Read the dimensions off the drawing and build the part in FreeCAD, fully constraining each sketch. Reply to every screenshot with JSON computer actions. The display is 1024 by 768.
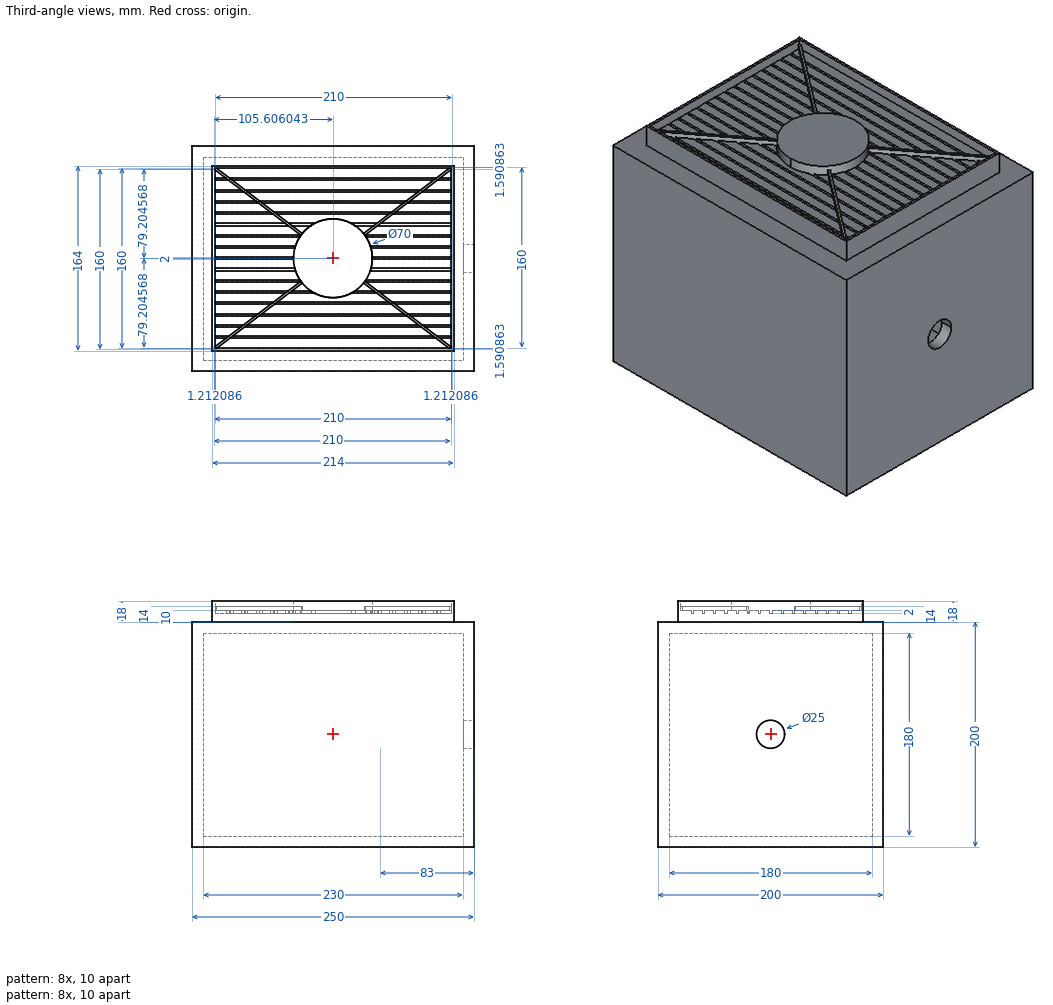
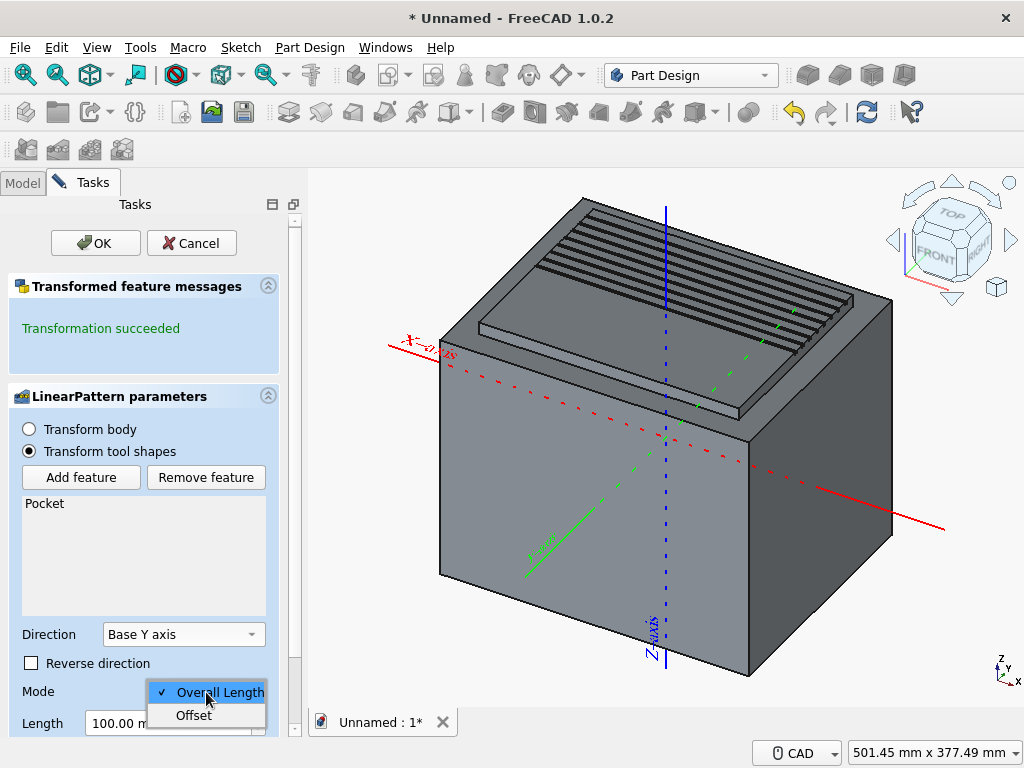
{"action": "left_click", "coordinate": [206, 716]}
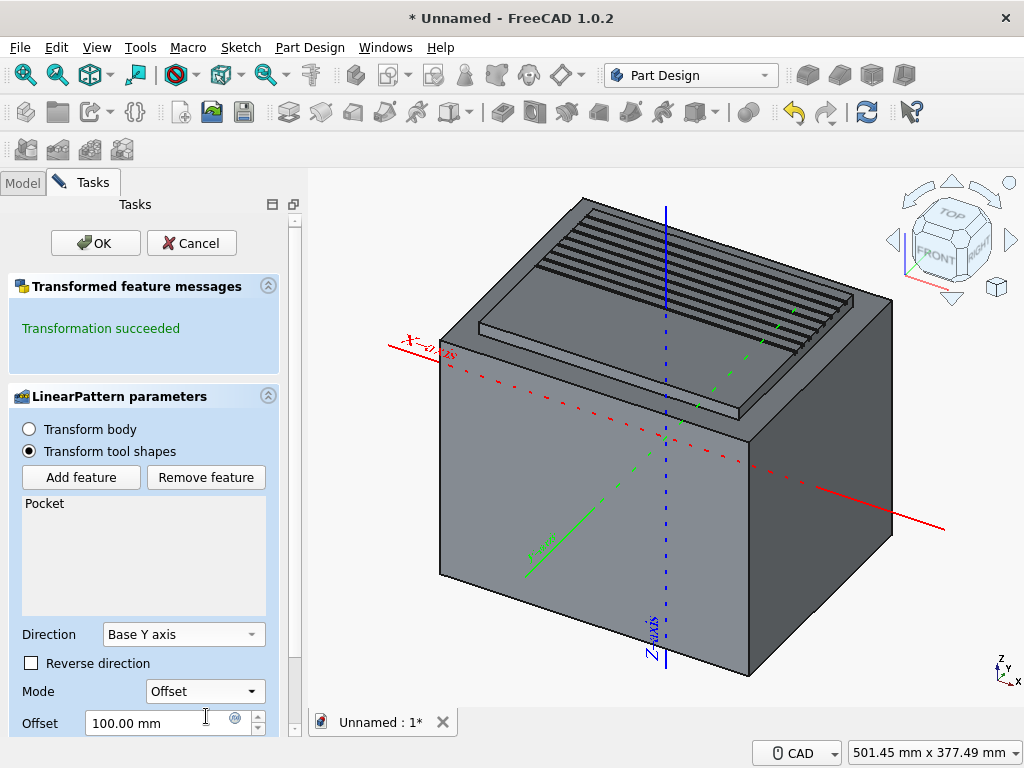
{"action": "triple_click", "coordinate": [168, 723]}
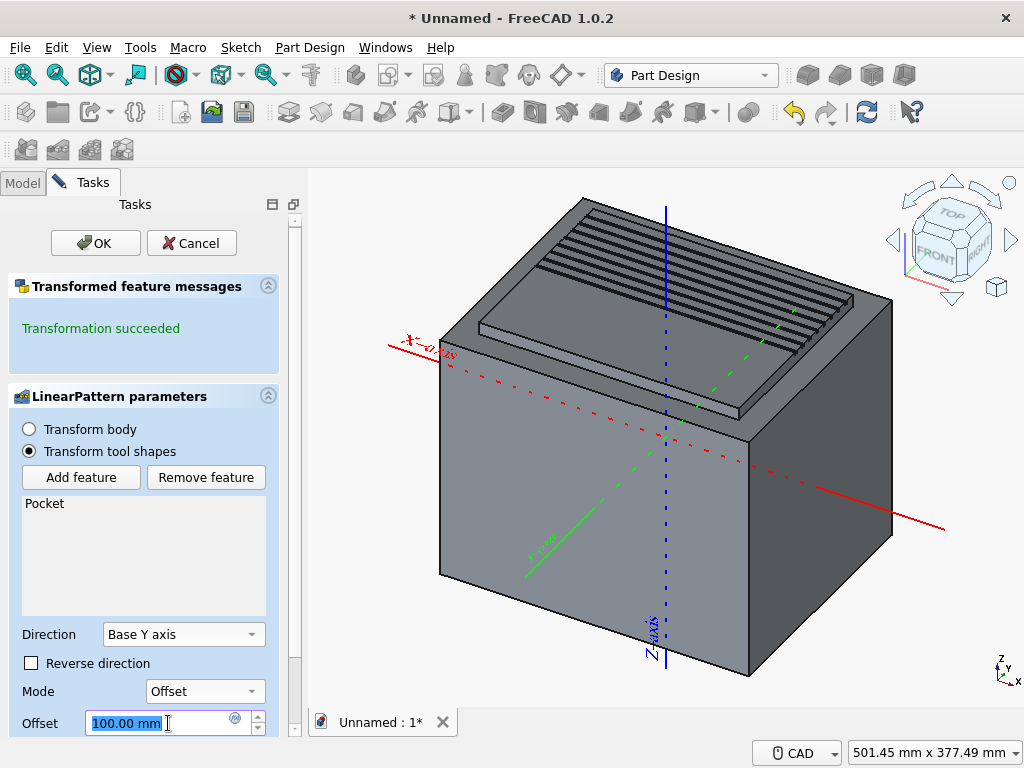
{"action": "type", "text": "10"}
{"action": "key", "text": "Tab"}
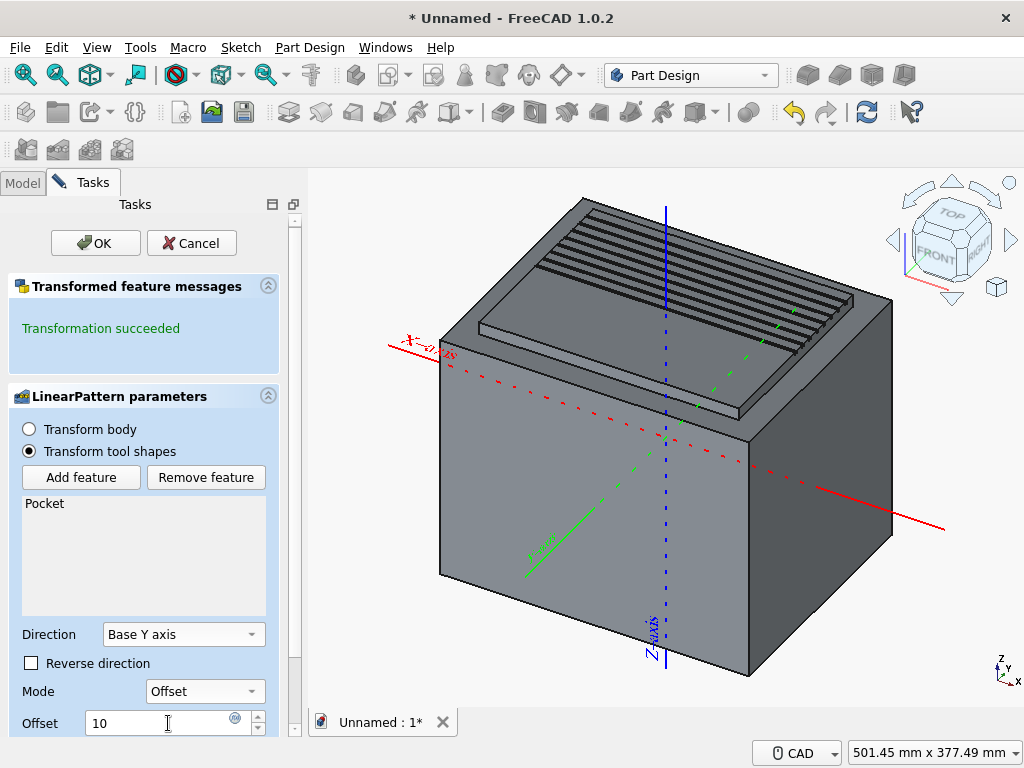
{"action": "scroll", "coordinate": [295, 475], "scroll_direction": "down", "scroll_amount": 2}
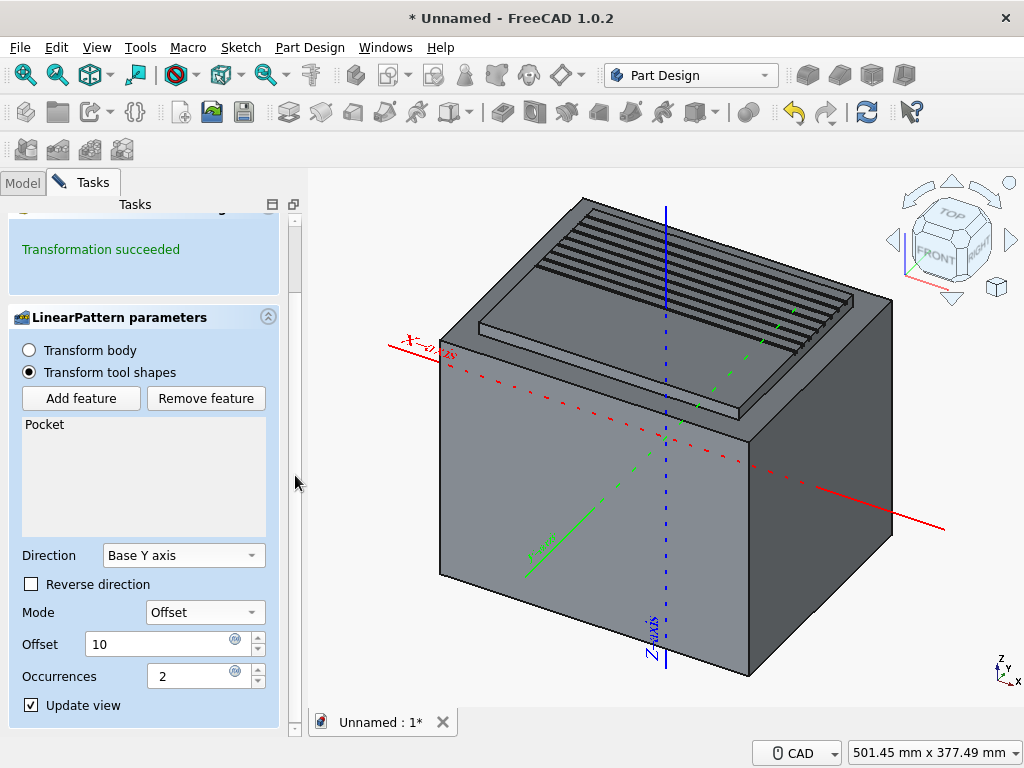
{"action": "triple_click", "coordinate": [198, 676]}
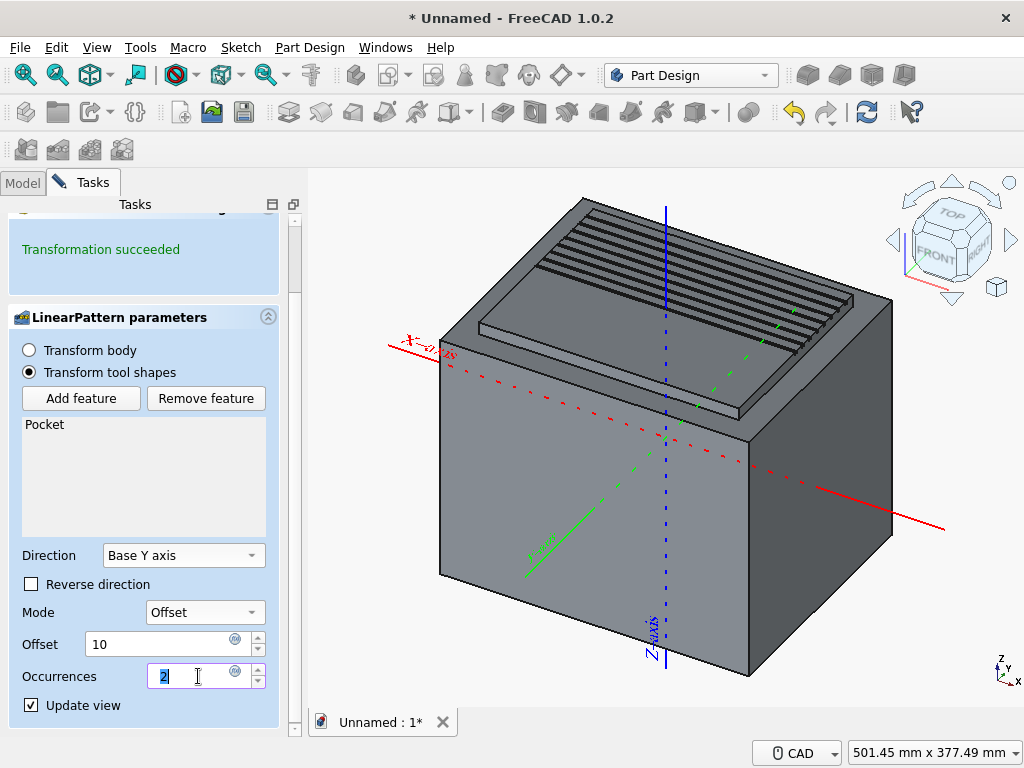
{"action": "type", "text": "8"}
{"action": "key", "text": "Tab"}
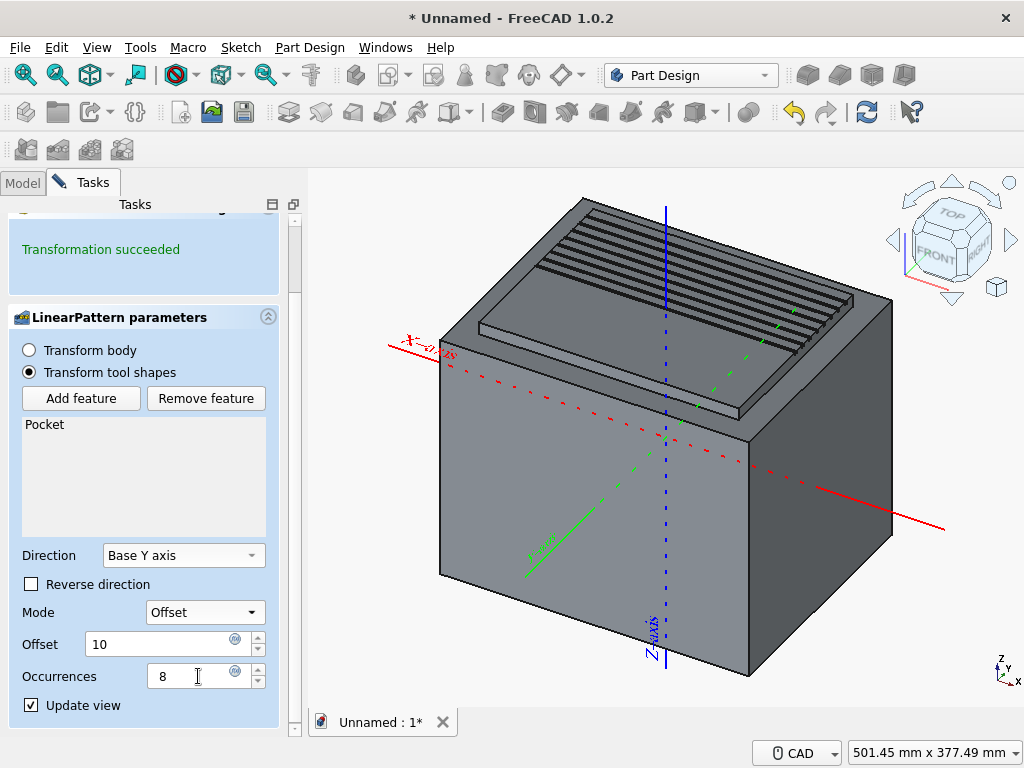
{"action": "left_click", "coordinate": [30, 584]}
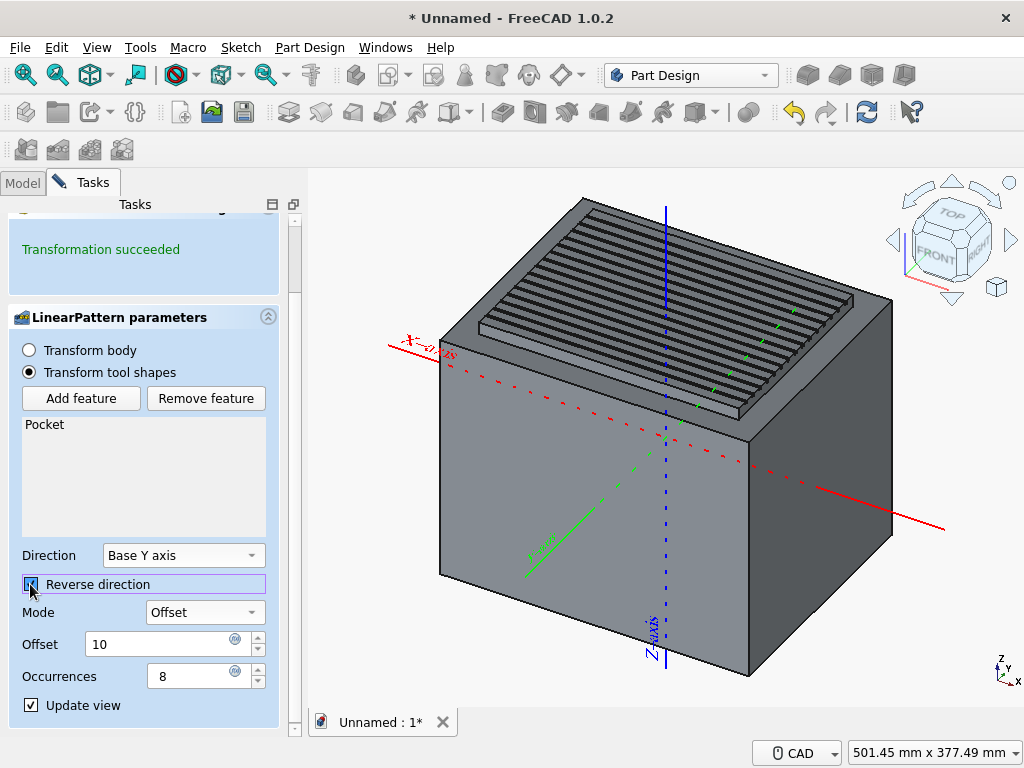
{"action": "scroll", "coordinate": [295, 475], "scroll_direction": "up", "scroll_amount": 3}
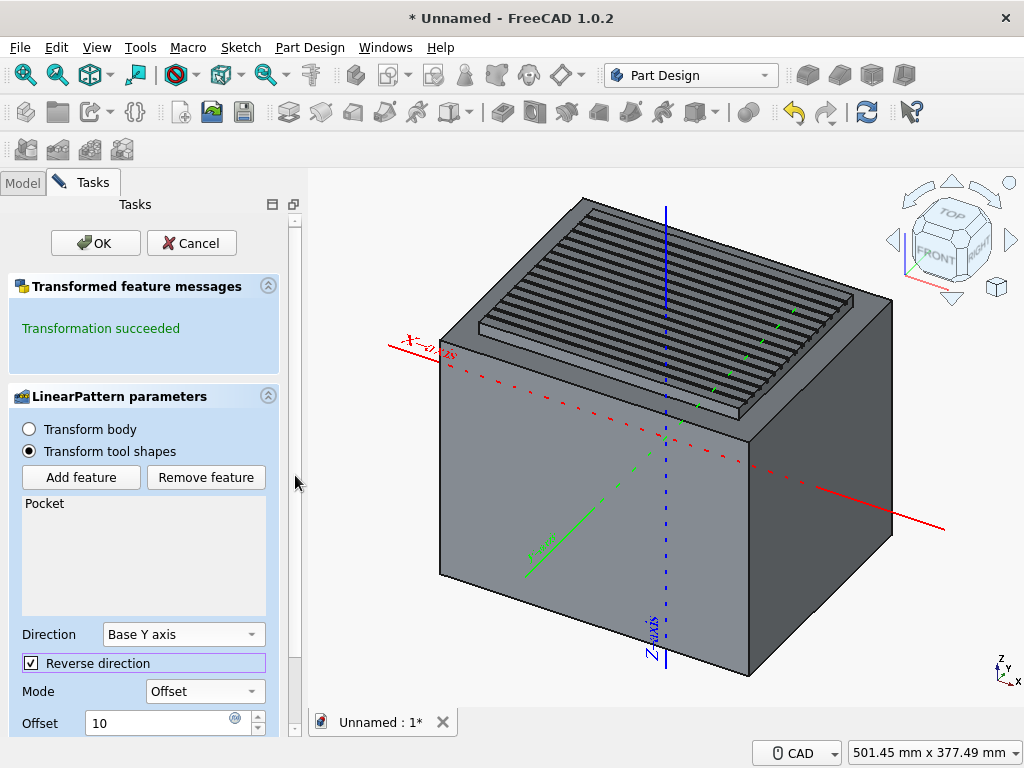
{"action": "left_click", "coordinate": [96, 243]}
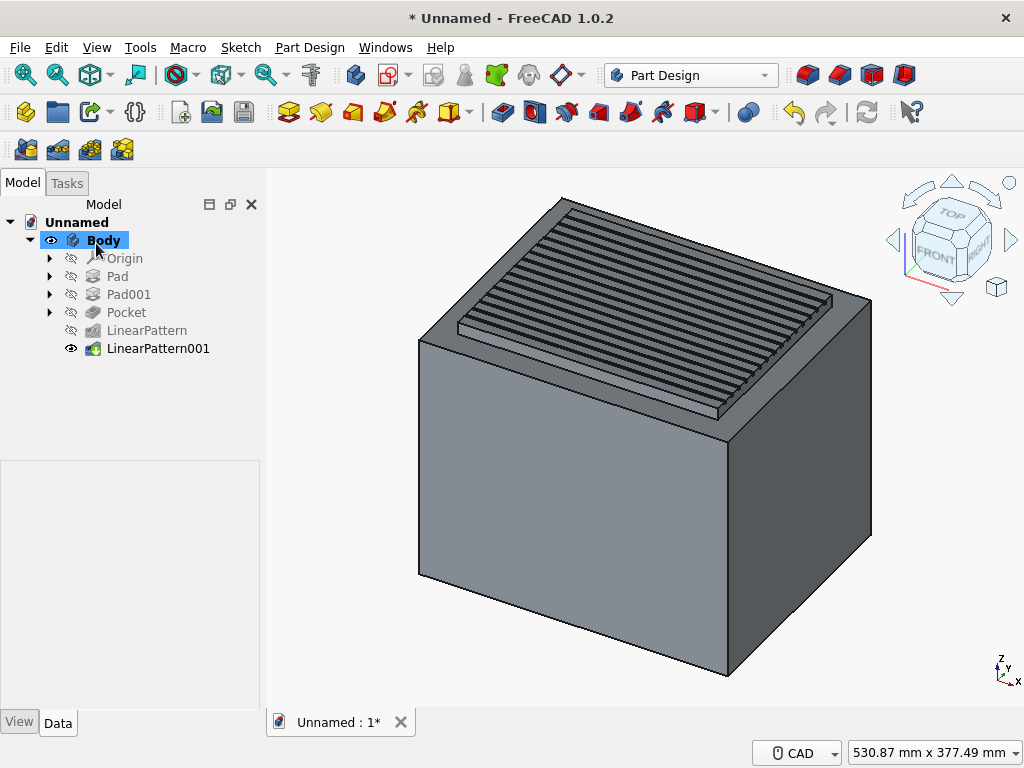
{"action": "left_click", "coordinate": [716, 424]}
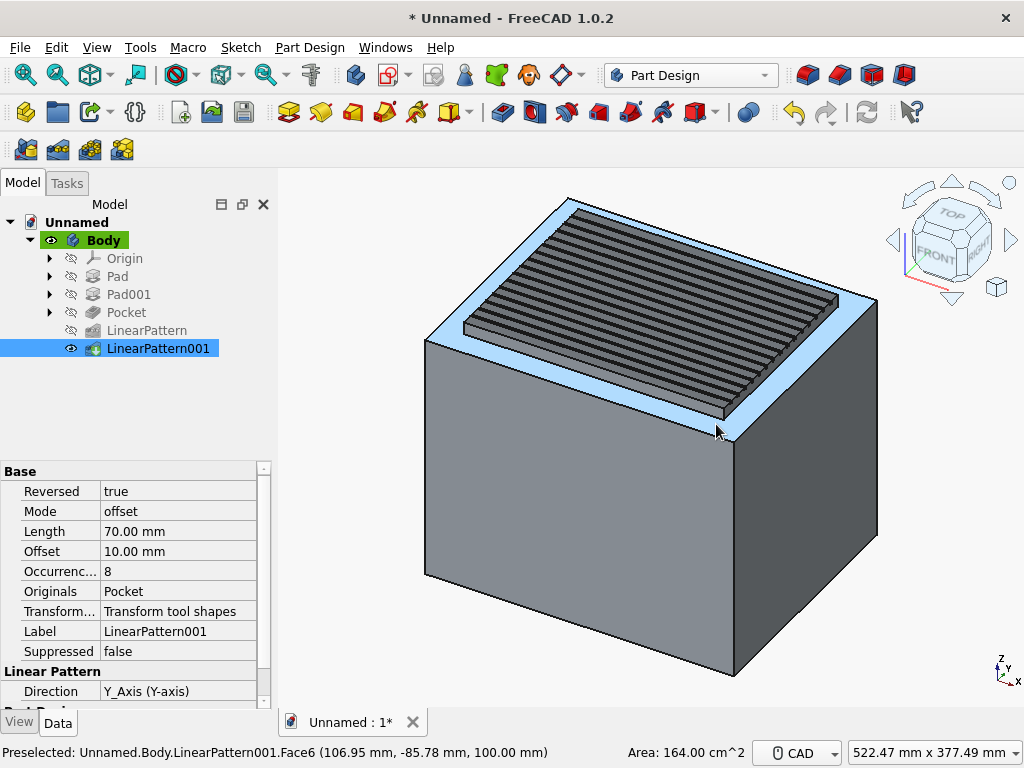
{"action": "left_click", "coordinate": [388, 76]}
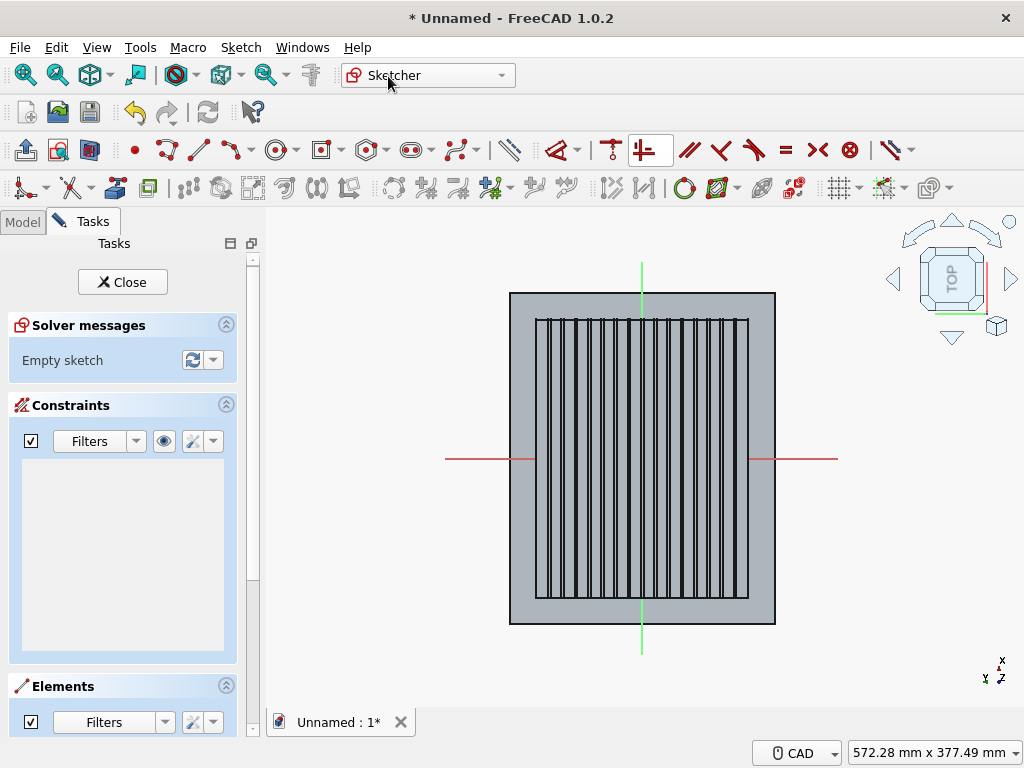
{"action": "left_click", "coordinate": [90, 150]}